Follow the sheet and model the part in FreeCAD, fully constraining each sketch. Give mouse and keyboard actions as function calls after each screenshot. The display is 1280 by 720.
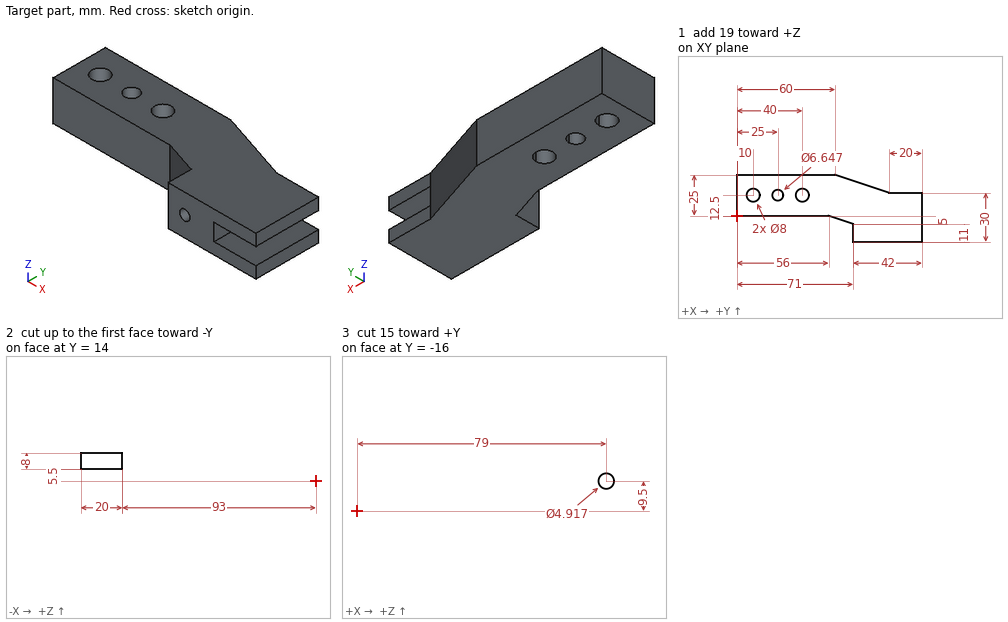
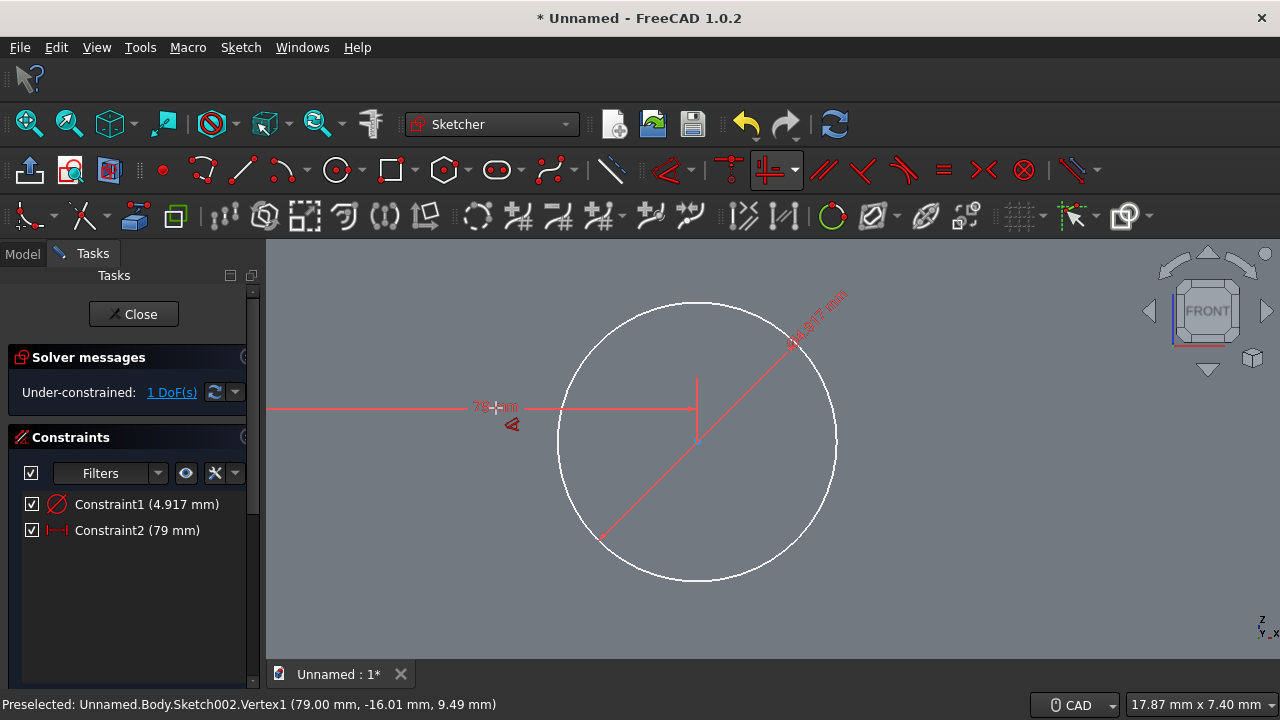
click(697, 442)
click(731, 536)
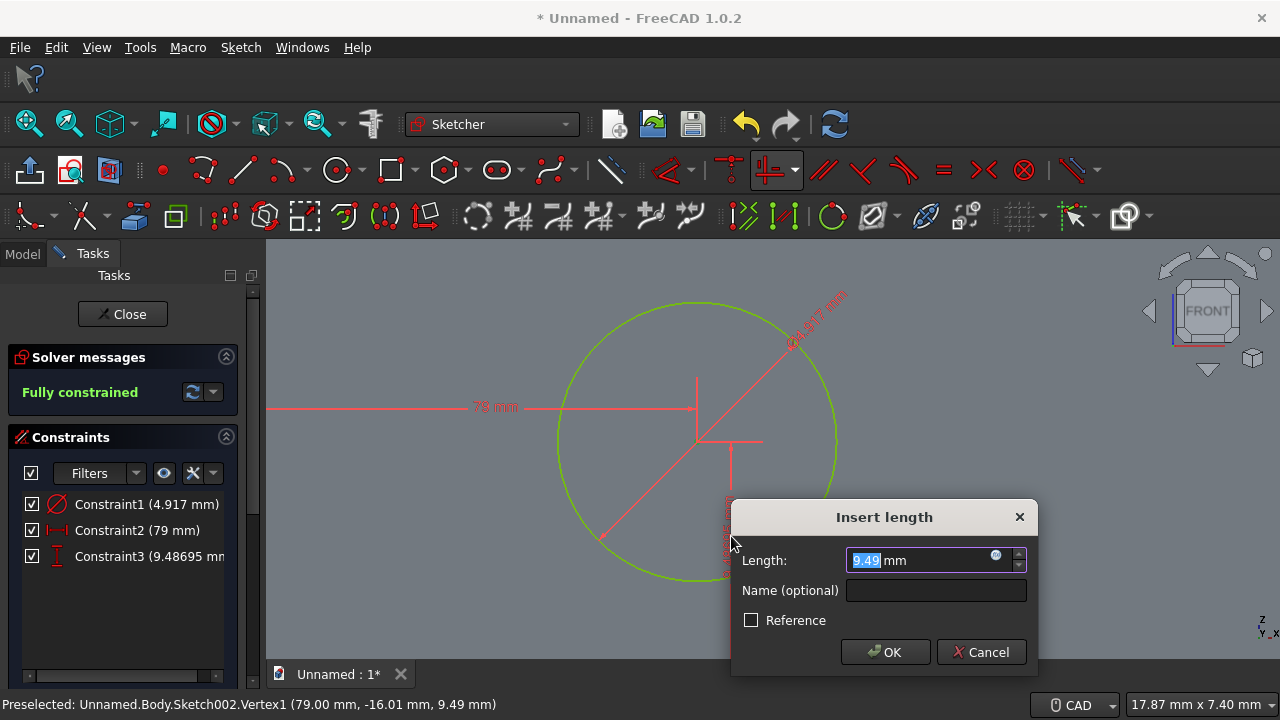
text(9.5)
key(Return)
key(Escape)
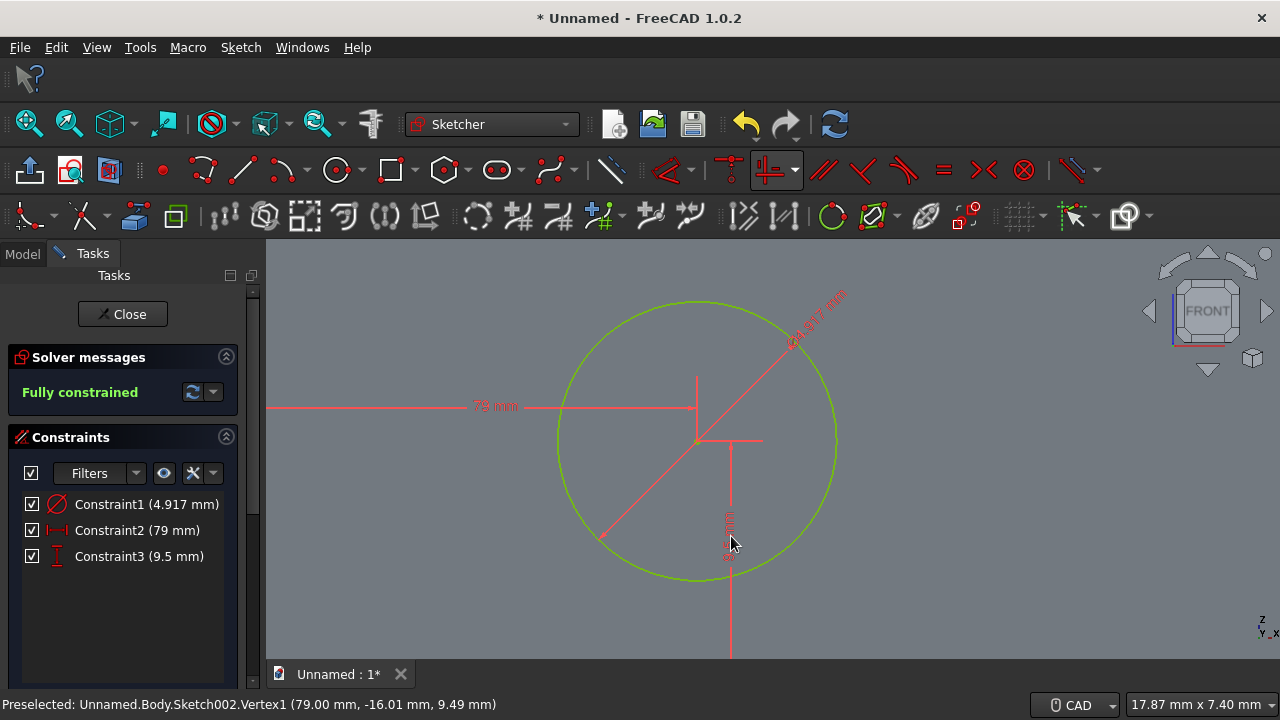
click(123, 314)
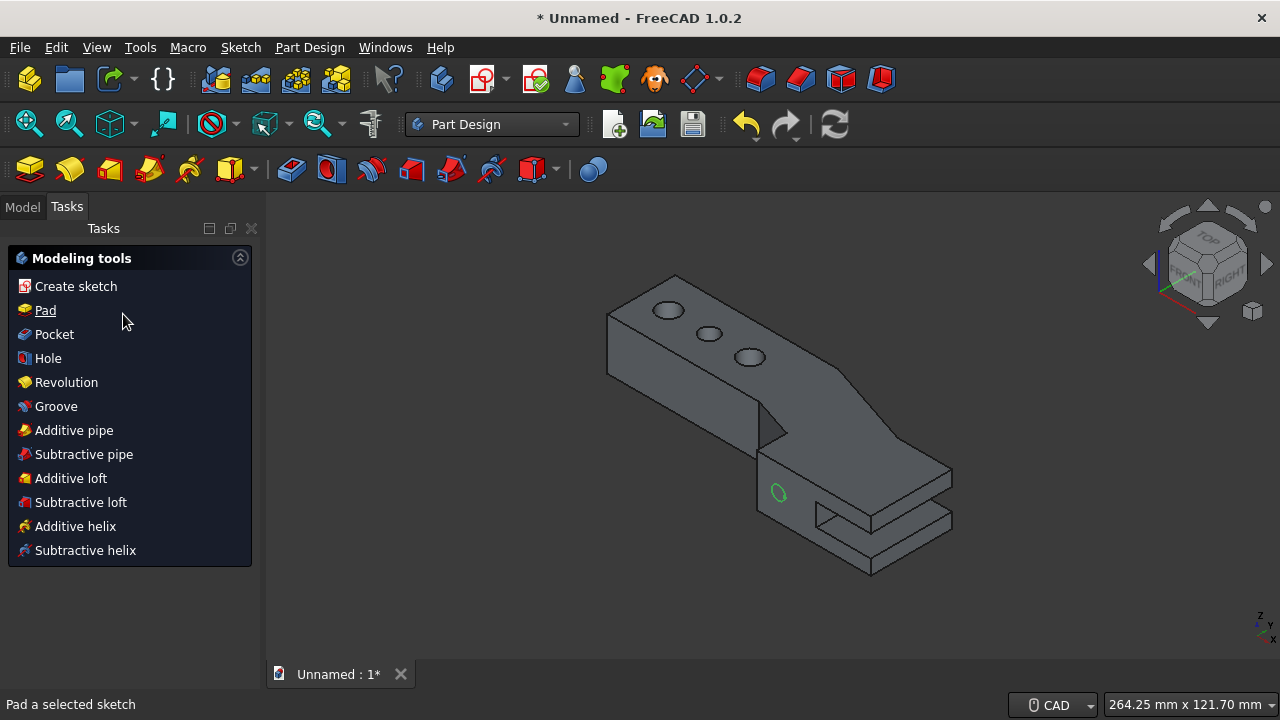
click(292, 170)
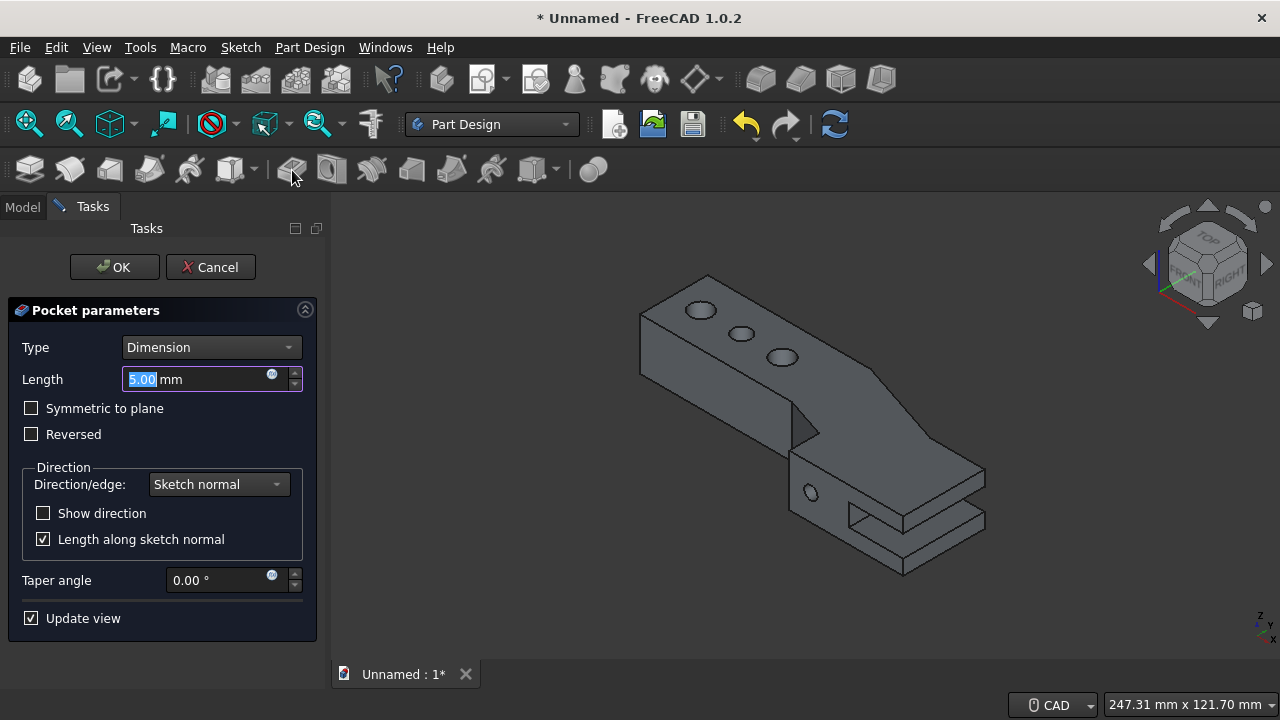
text(15)
key(Tab)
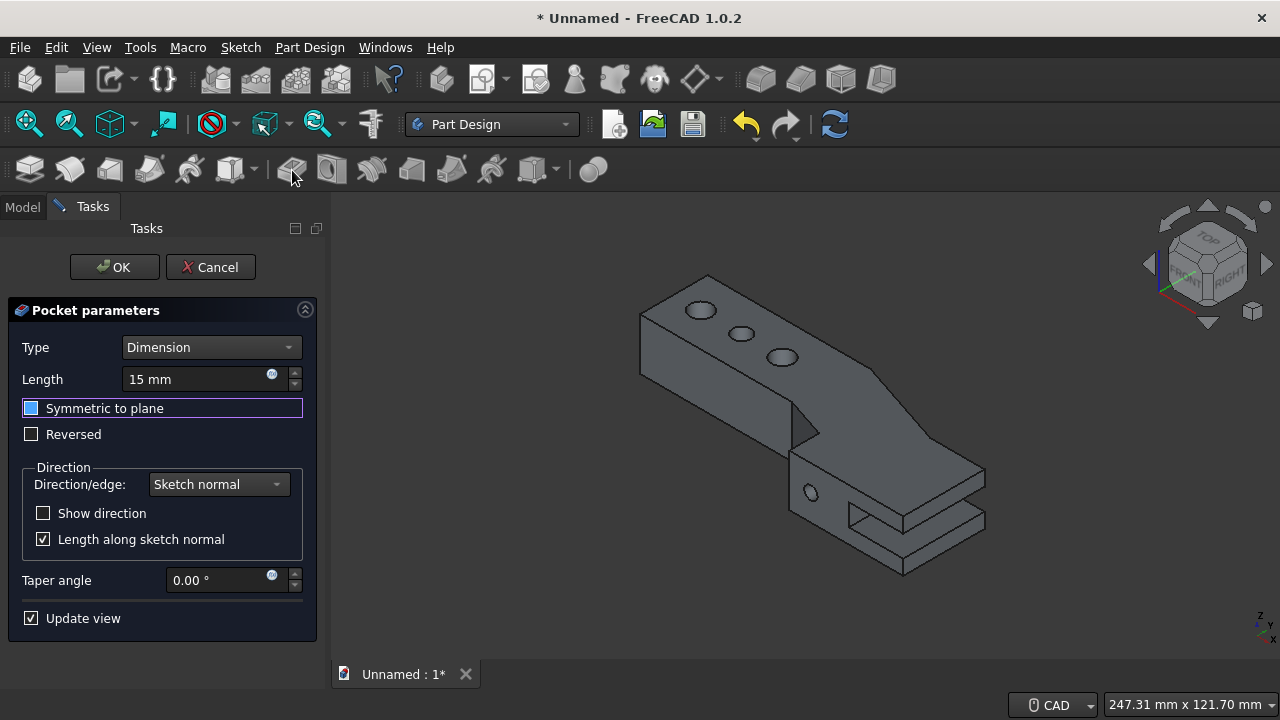
click(115, 267)